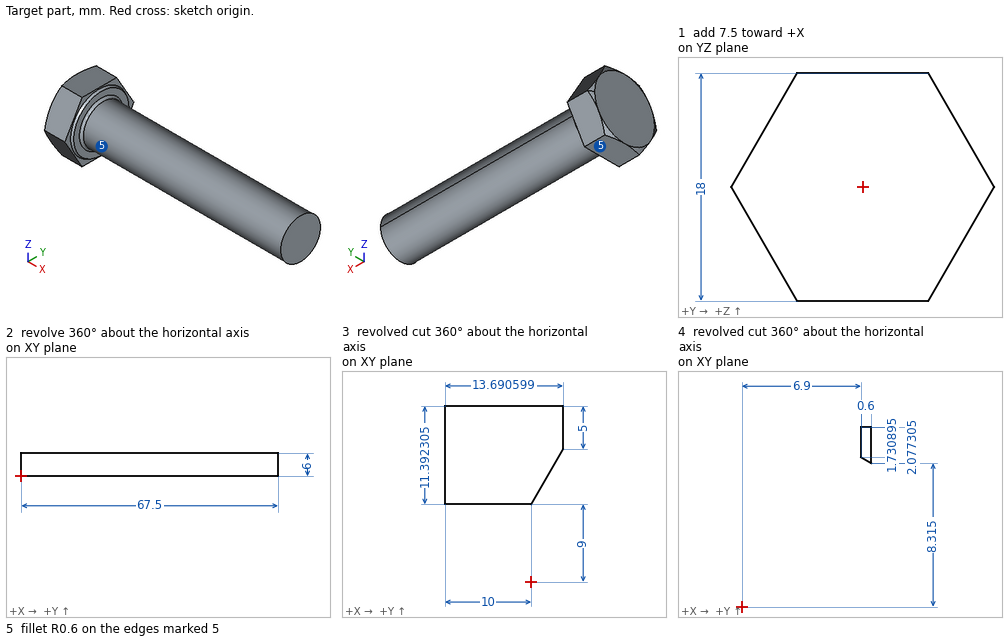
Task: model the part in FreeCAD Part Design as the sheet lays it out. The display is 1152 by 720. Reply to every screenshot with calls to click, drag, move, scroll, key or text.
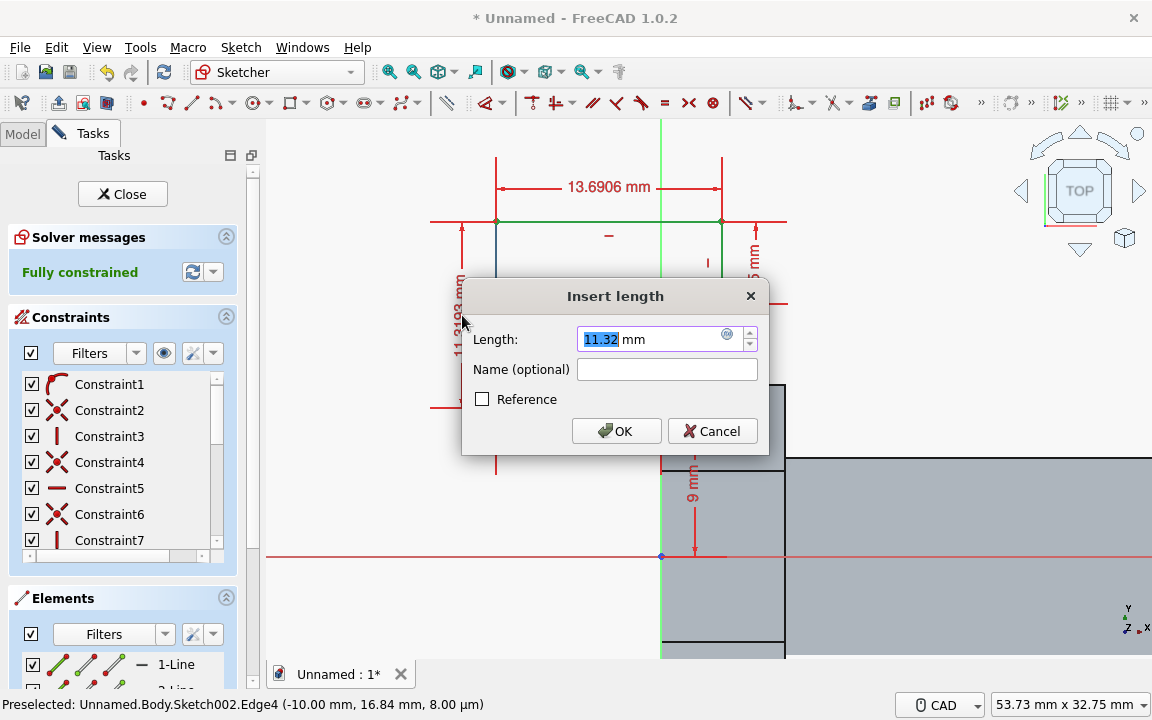
text(11.392305)
key(Return)
key(Escape)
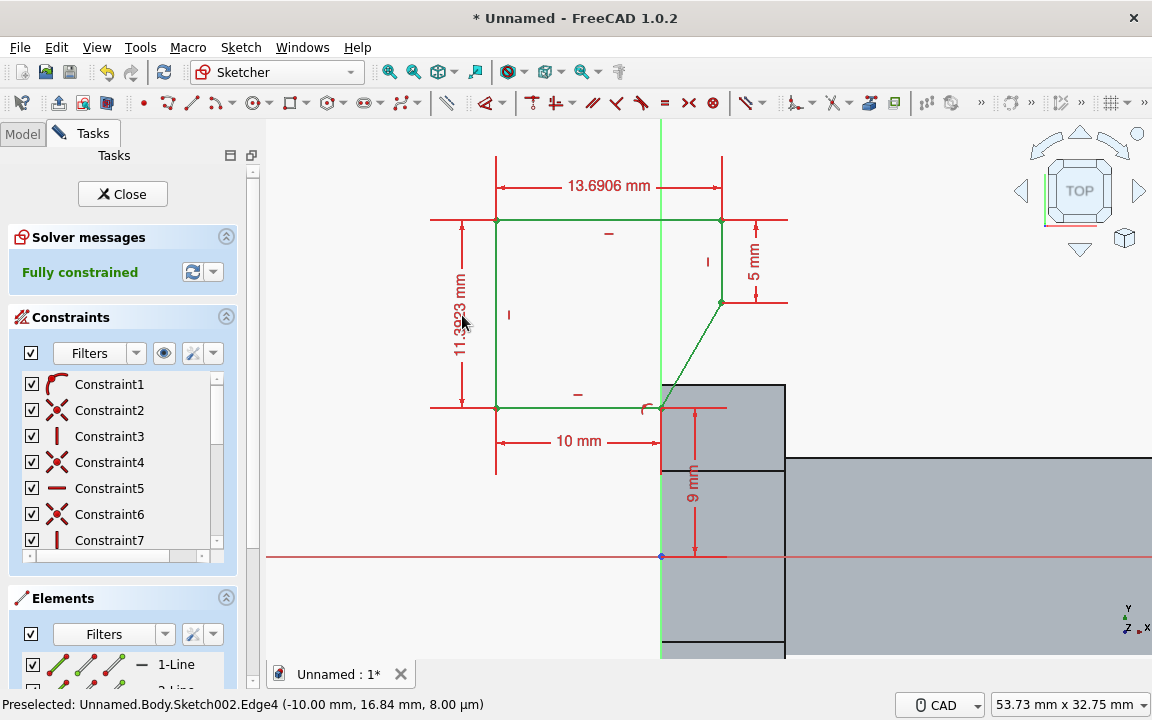
click(123, 194)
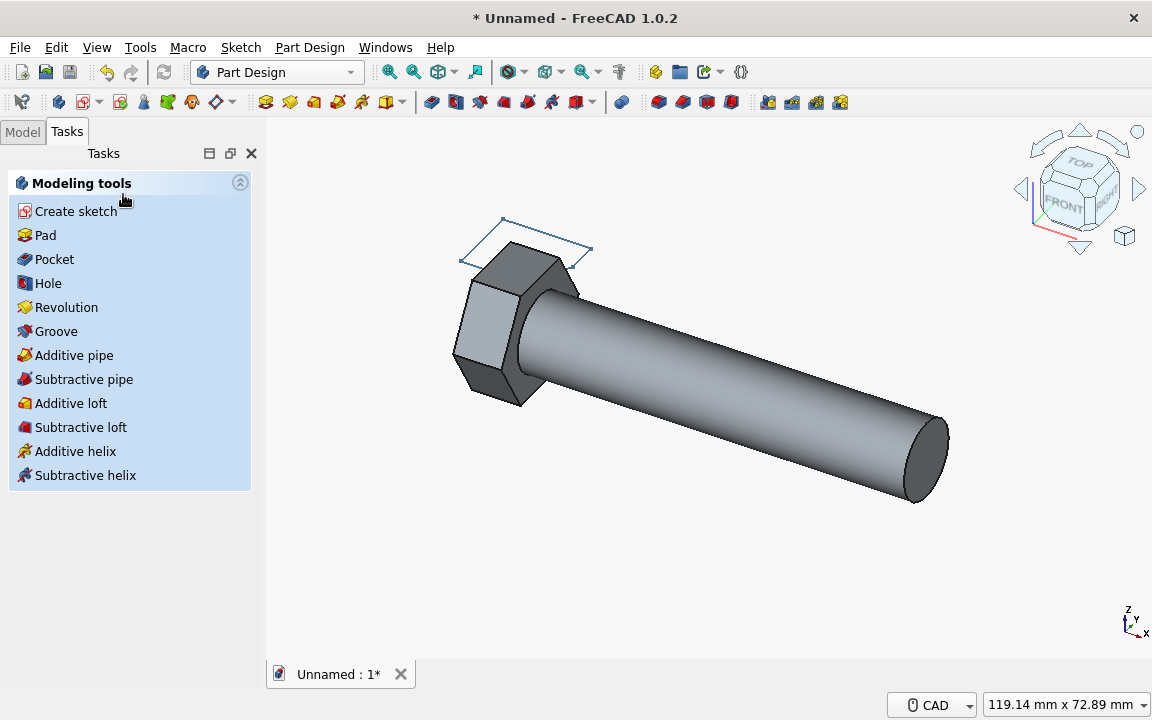
click(480, 102)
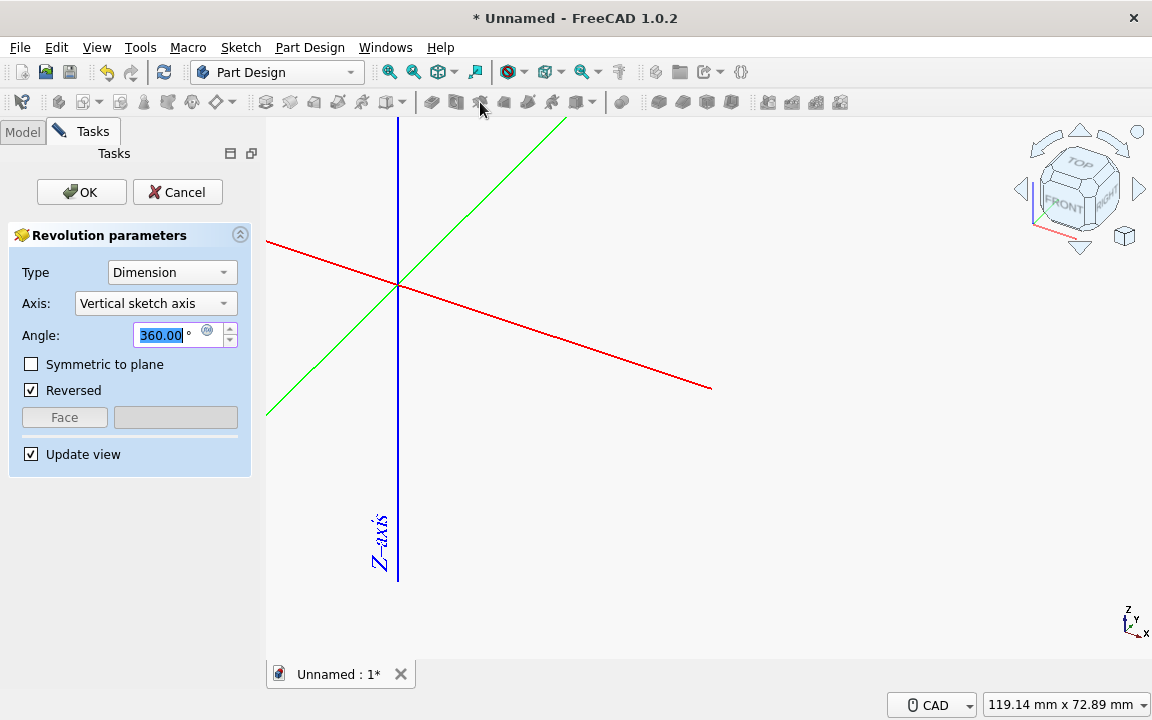
click(156, 304)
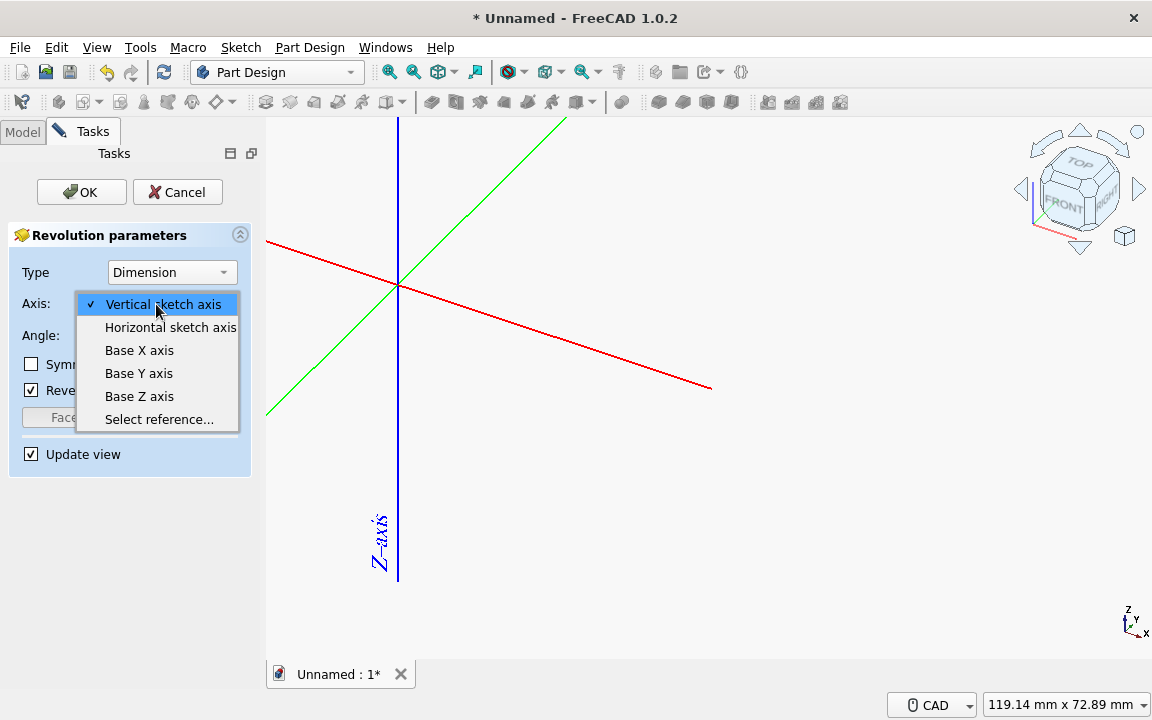
click(156, 328)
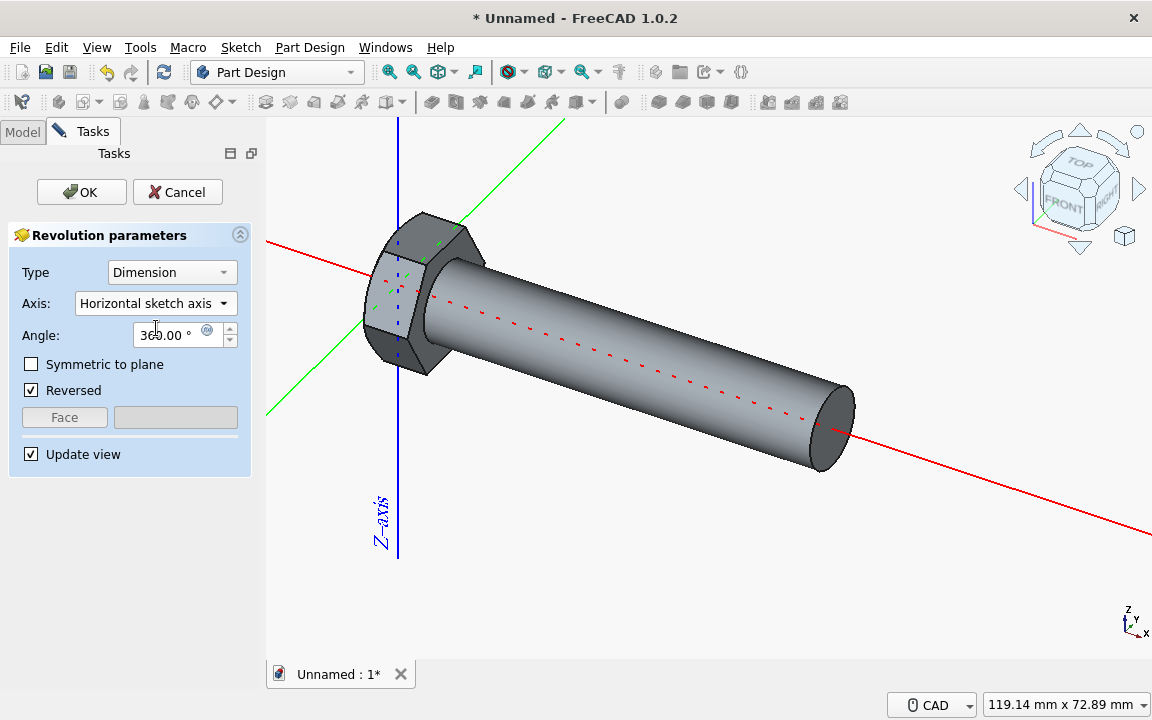
click(82, 192)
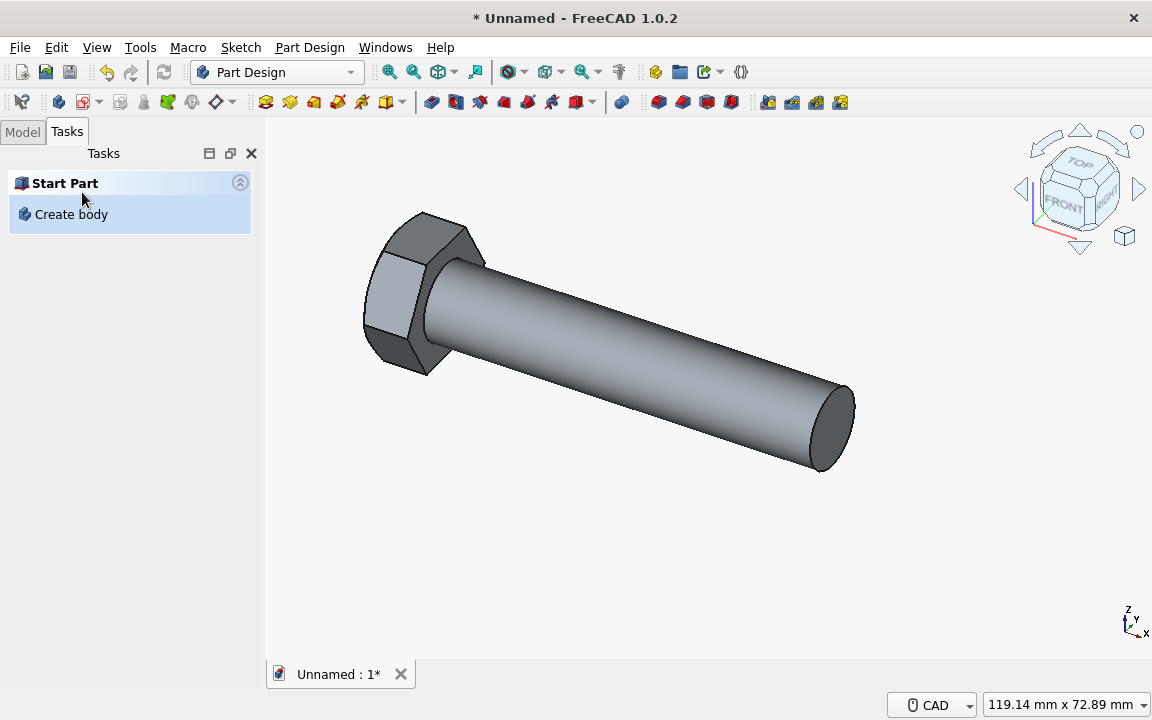
click(84, 102)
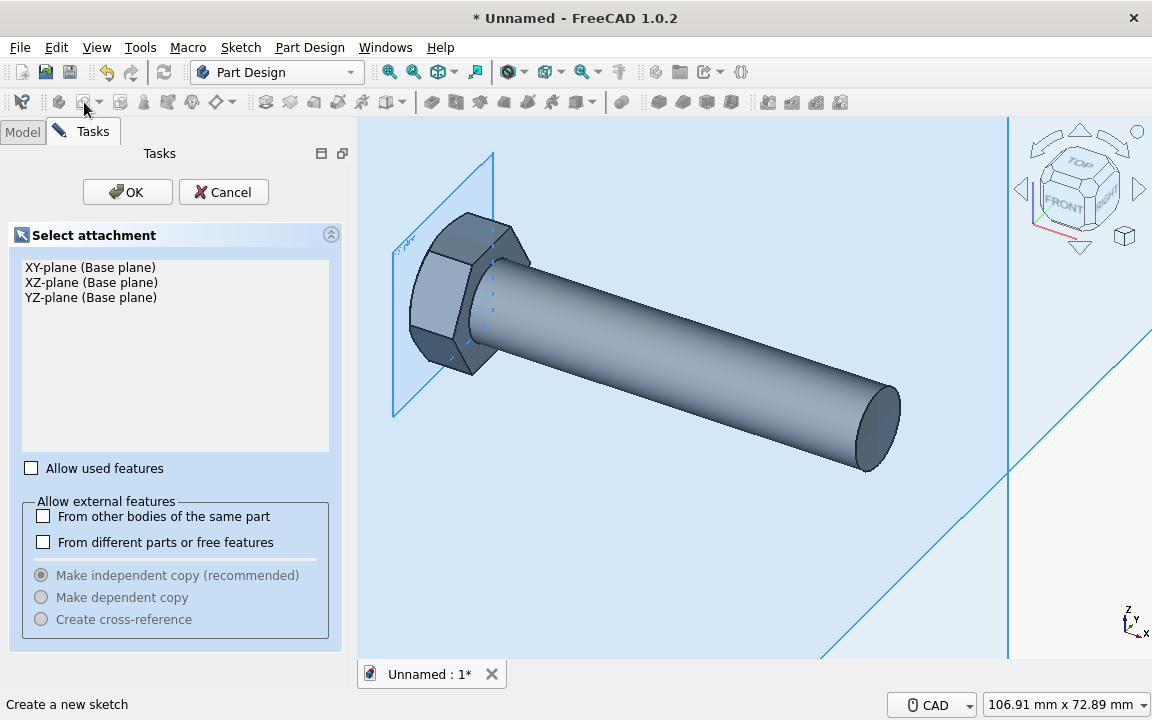
click(82, 268)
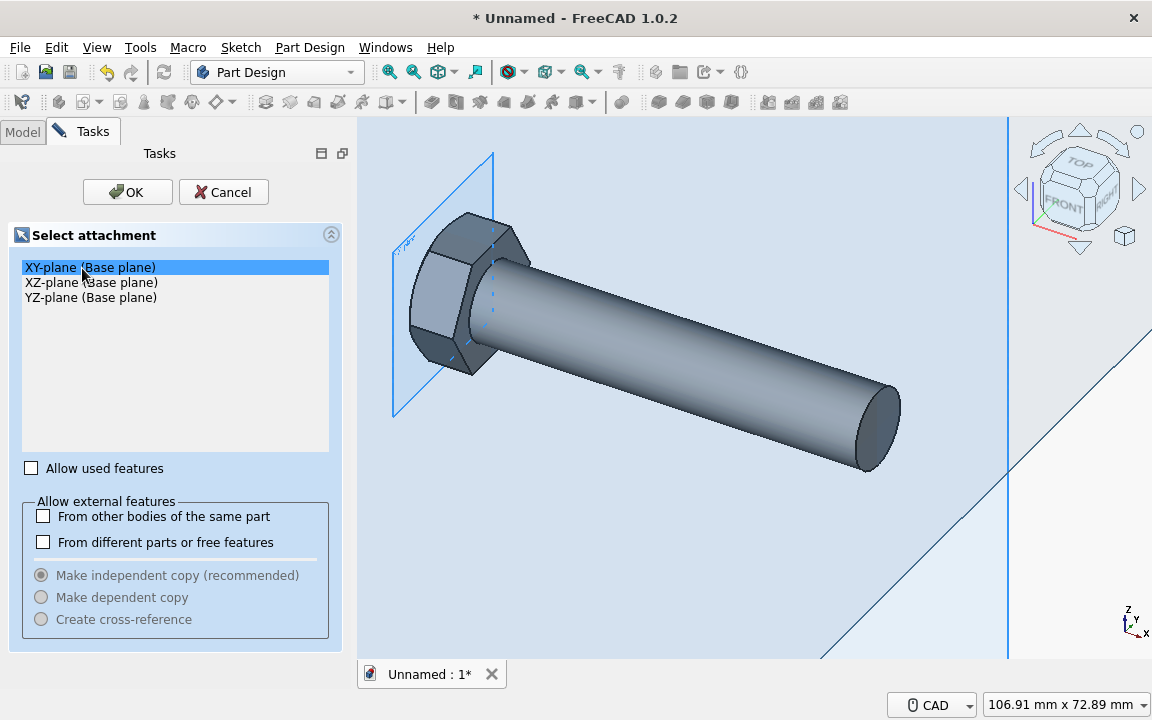
click(128, 192)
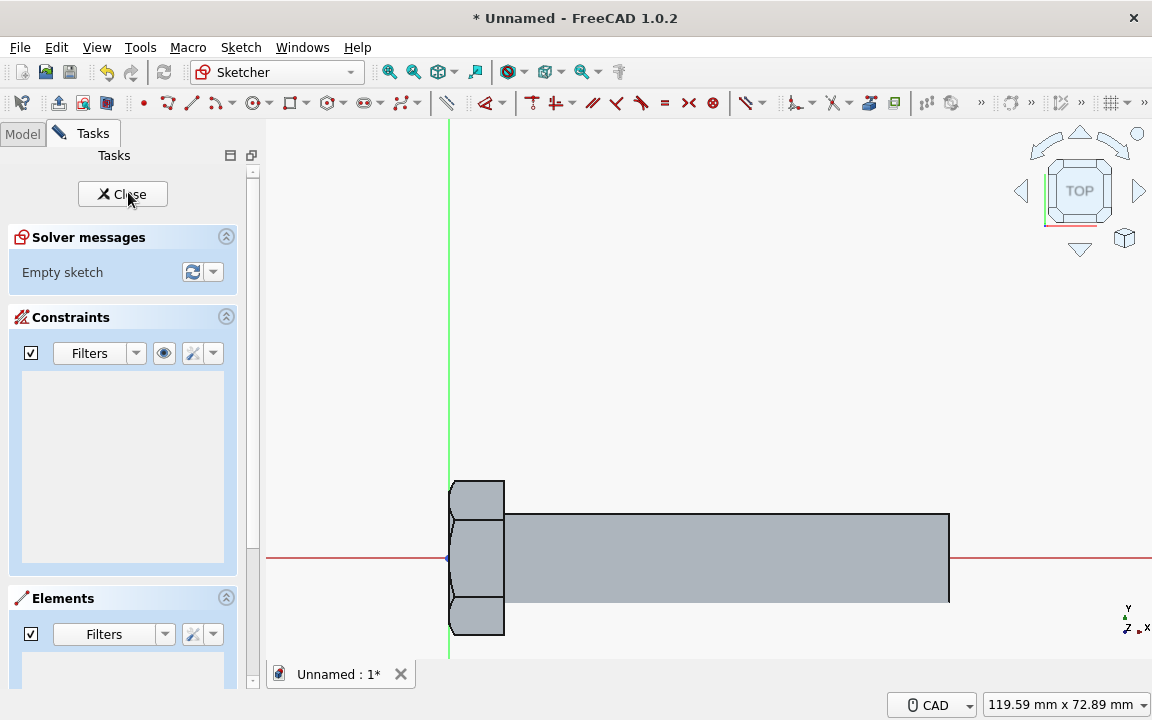
click(108, 104)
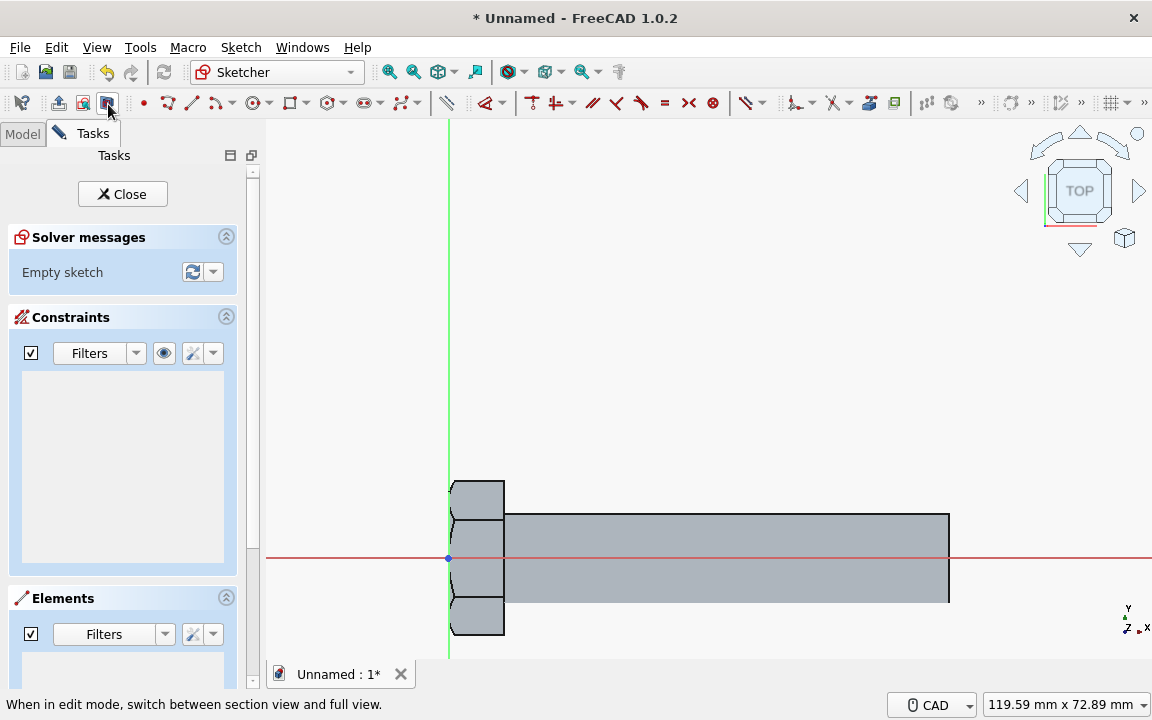
scroll(495, 494, up, 15)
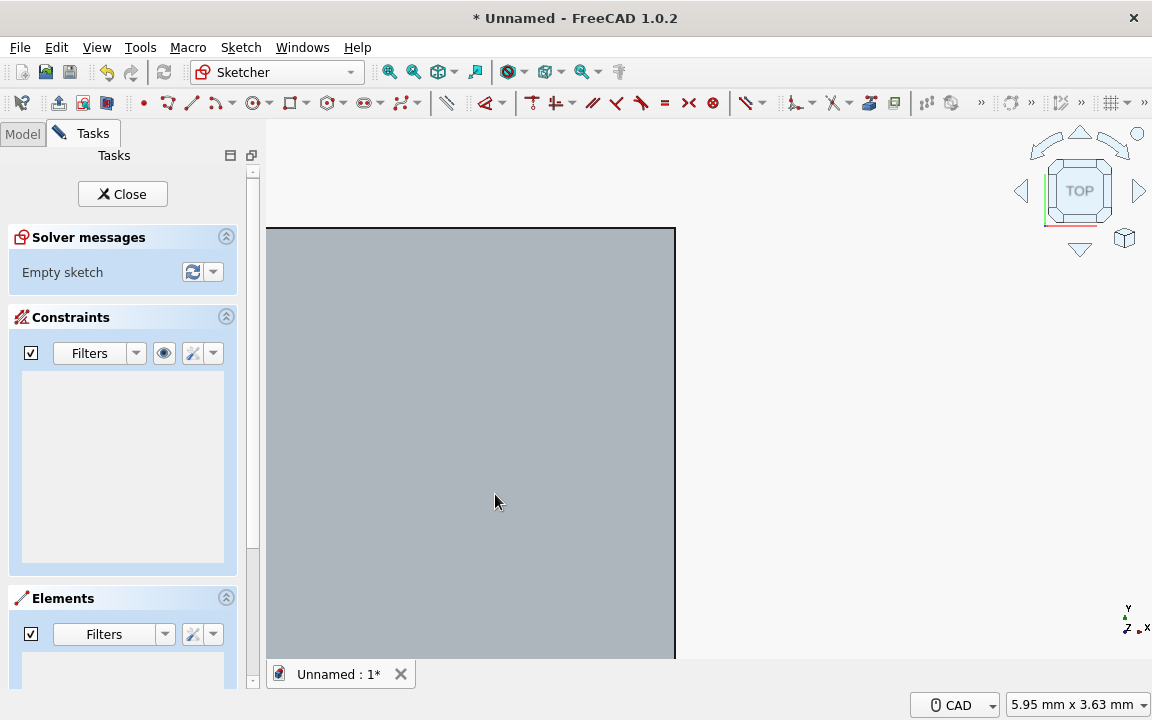
click(168, 104)